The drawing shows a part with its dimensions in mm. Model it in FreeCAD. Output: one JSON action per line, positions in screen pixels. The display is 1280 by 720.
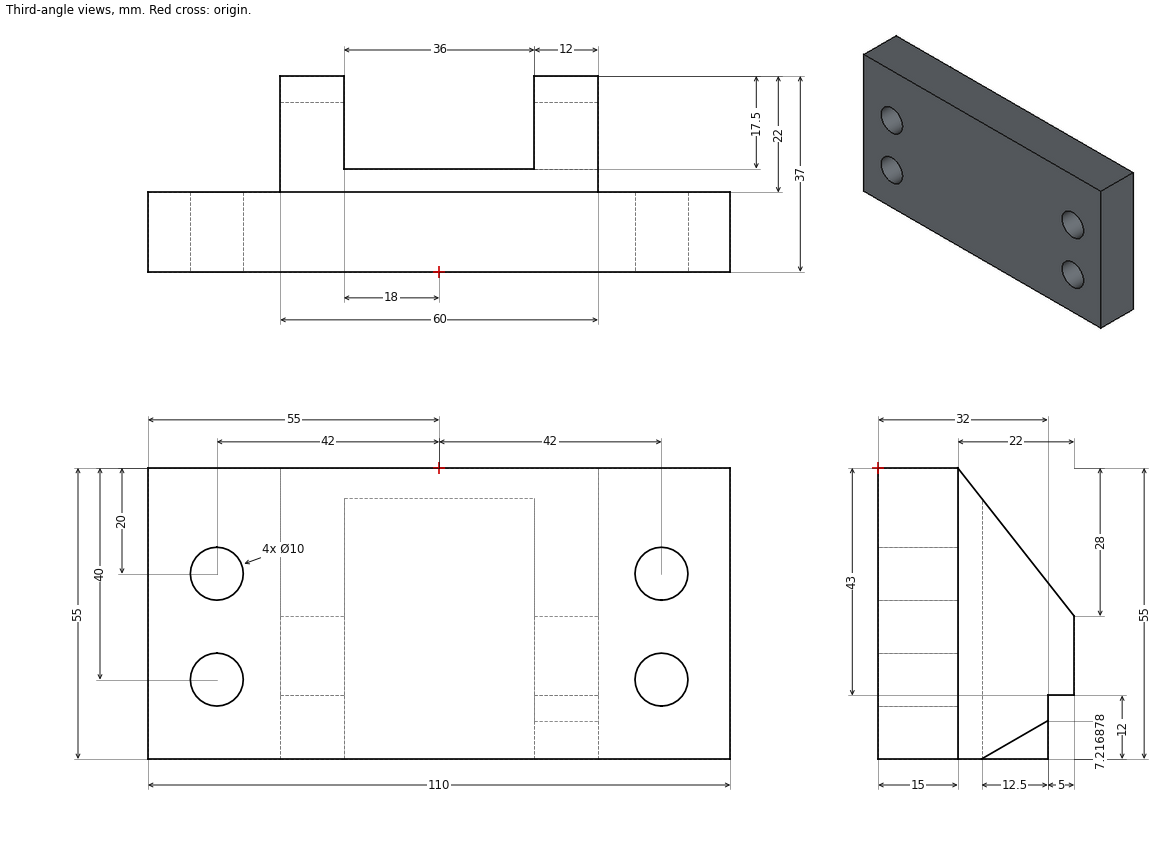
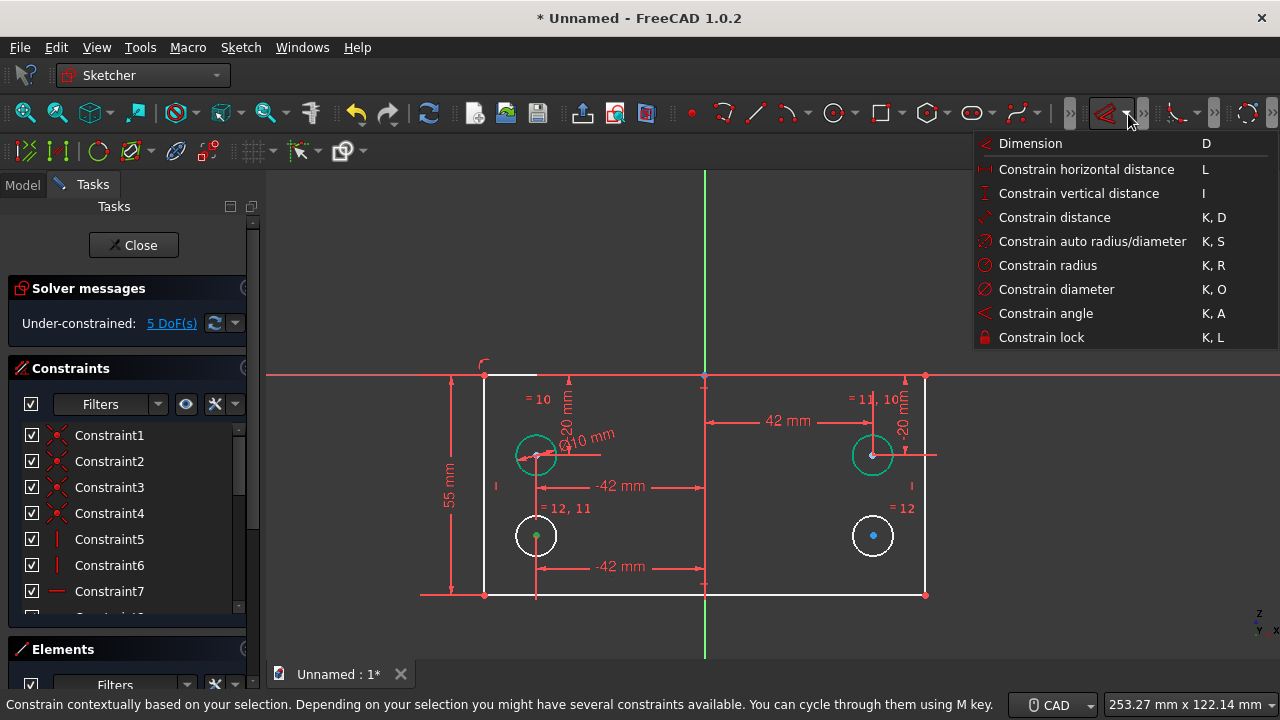
{"action": "left_click", "coordinate": [1126, 193]}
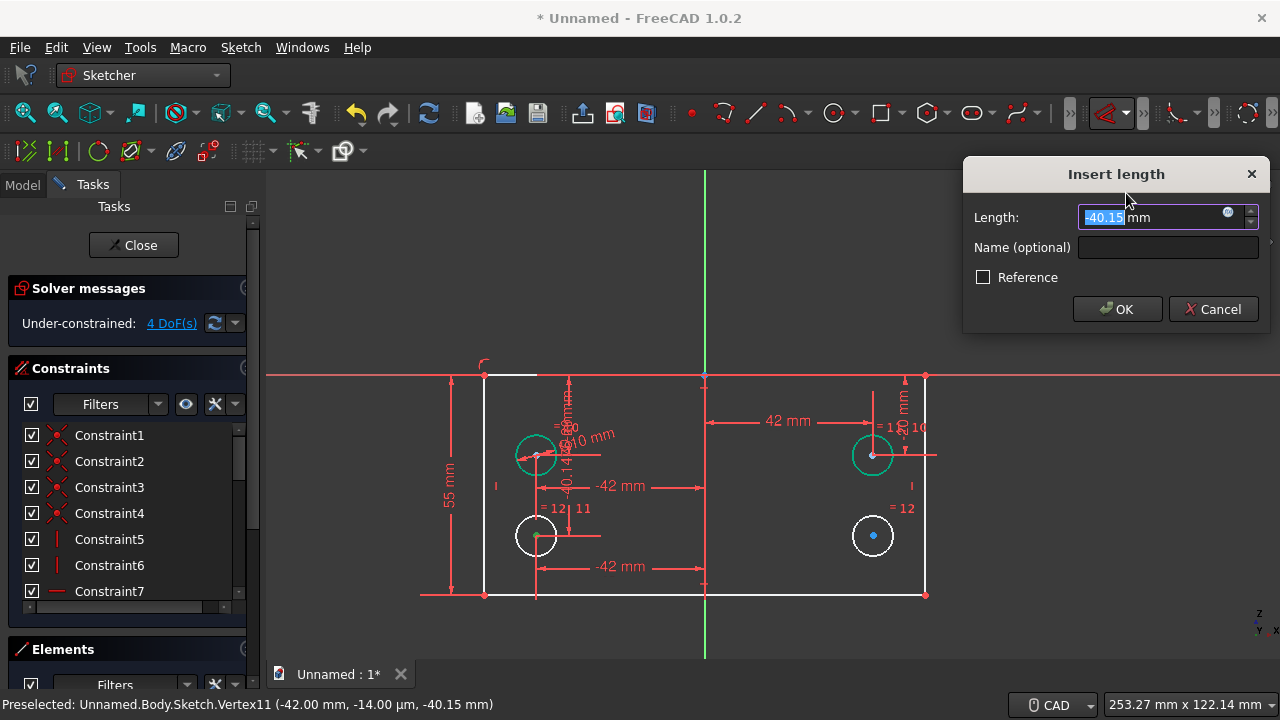
{"action": "type", "text": "-40"}
{"action": "key", "text": "Return"}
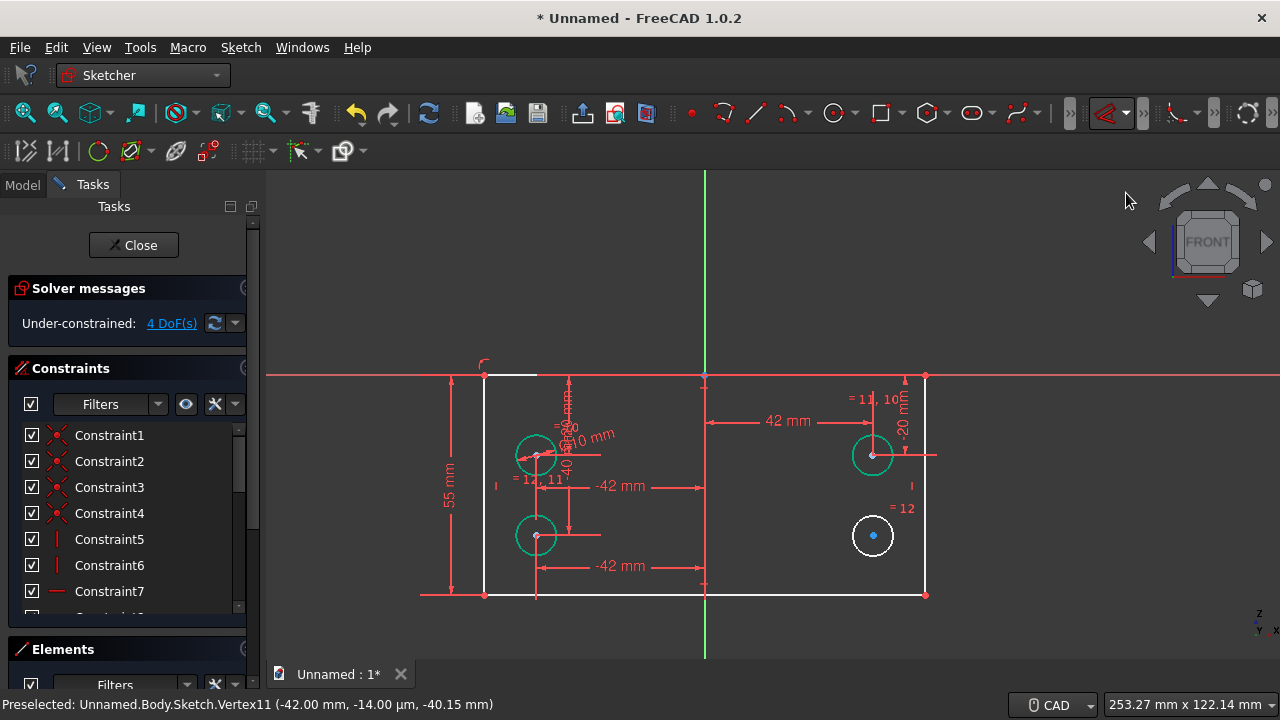
{"action": "left_click", "coordinate": [873, 536]}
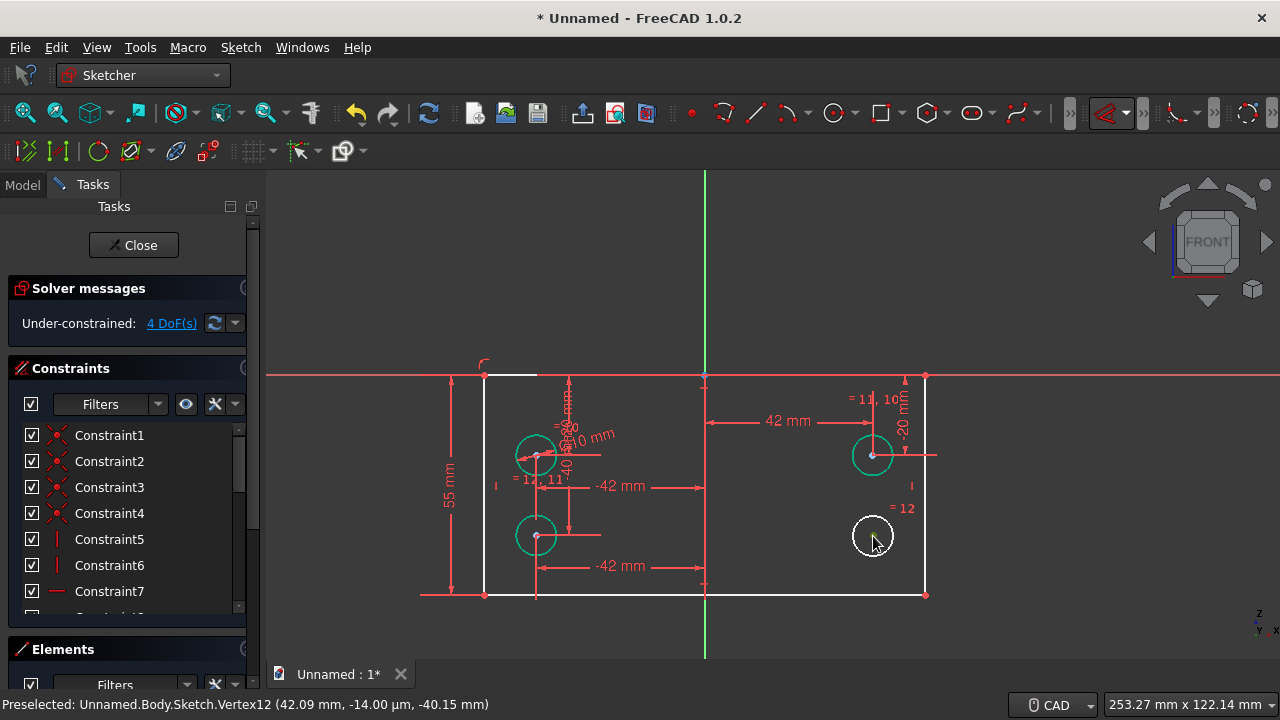
{"action": "key", "text": "l"}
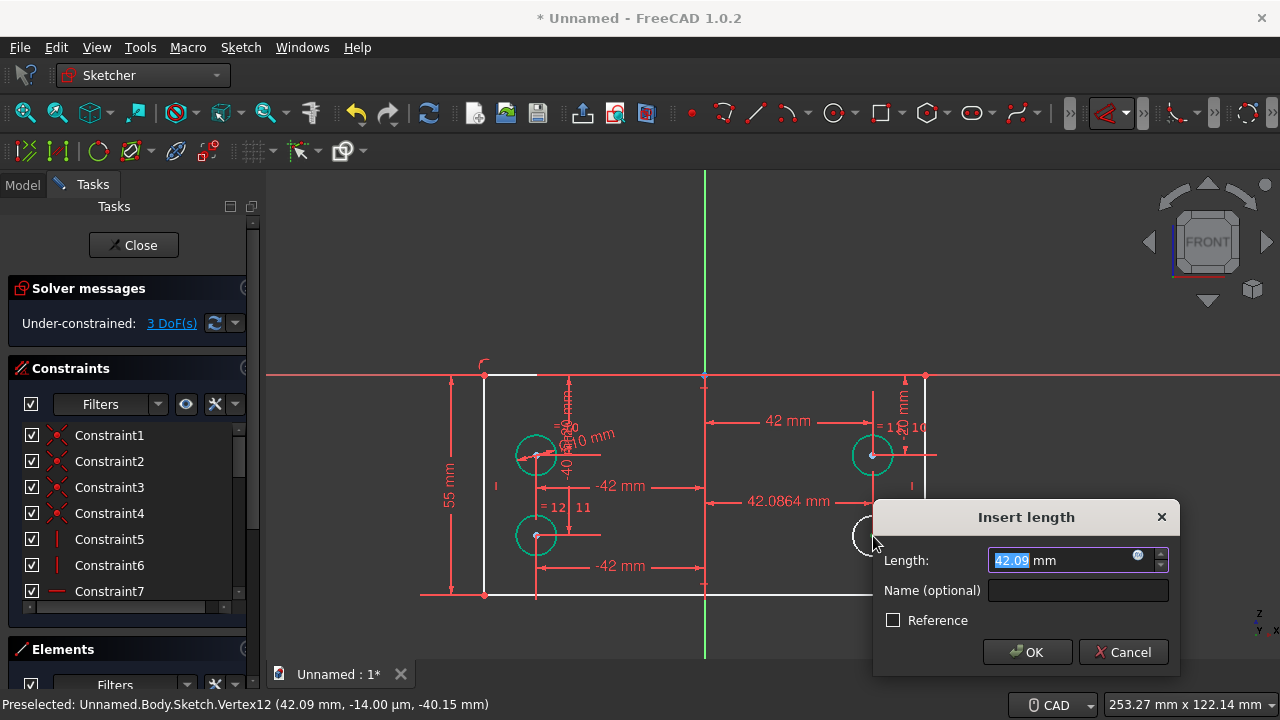
{"action": "type", "text": "42"}
{"action": "key", "text": "Return"}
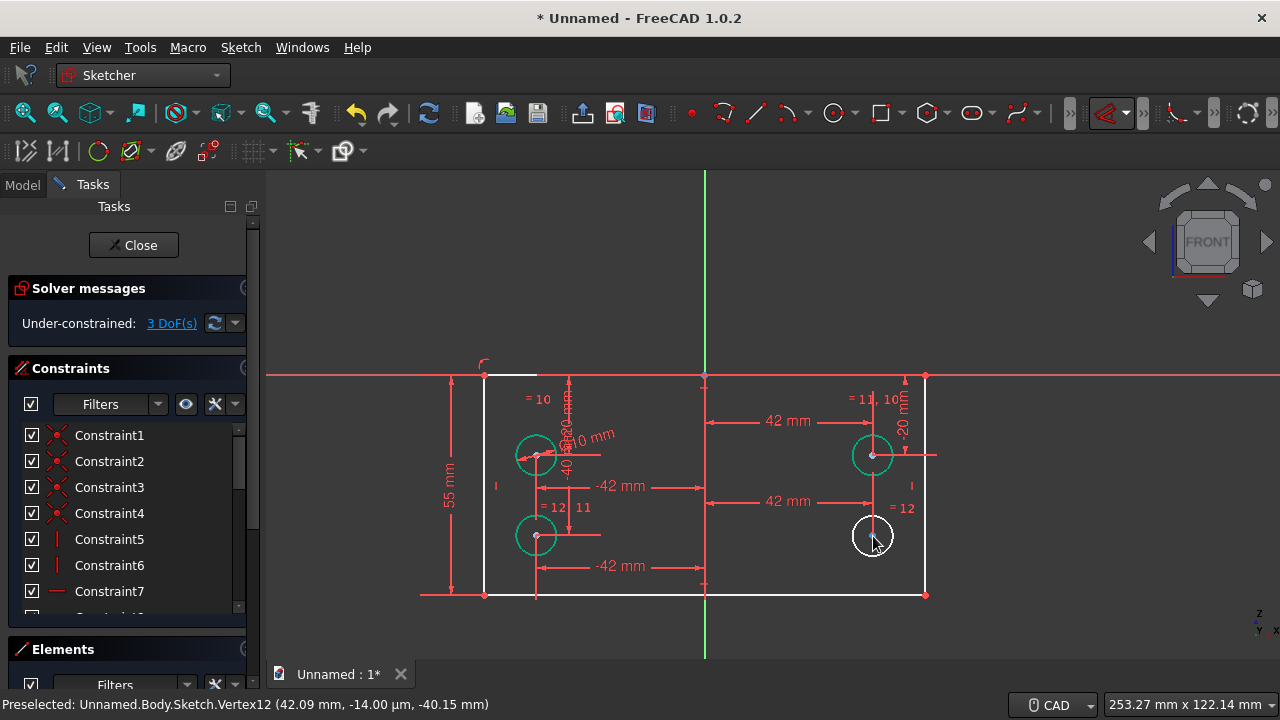
{"action": "left_click", "coordinate": [873, 536]}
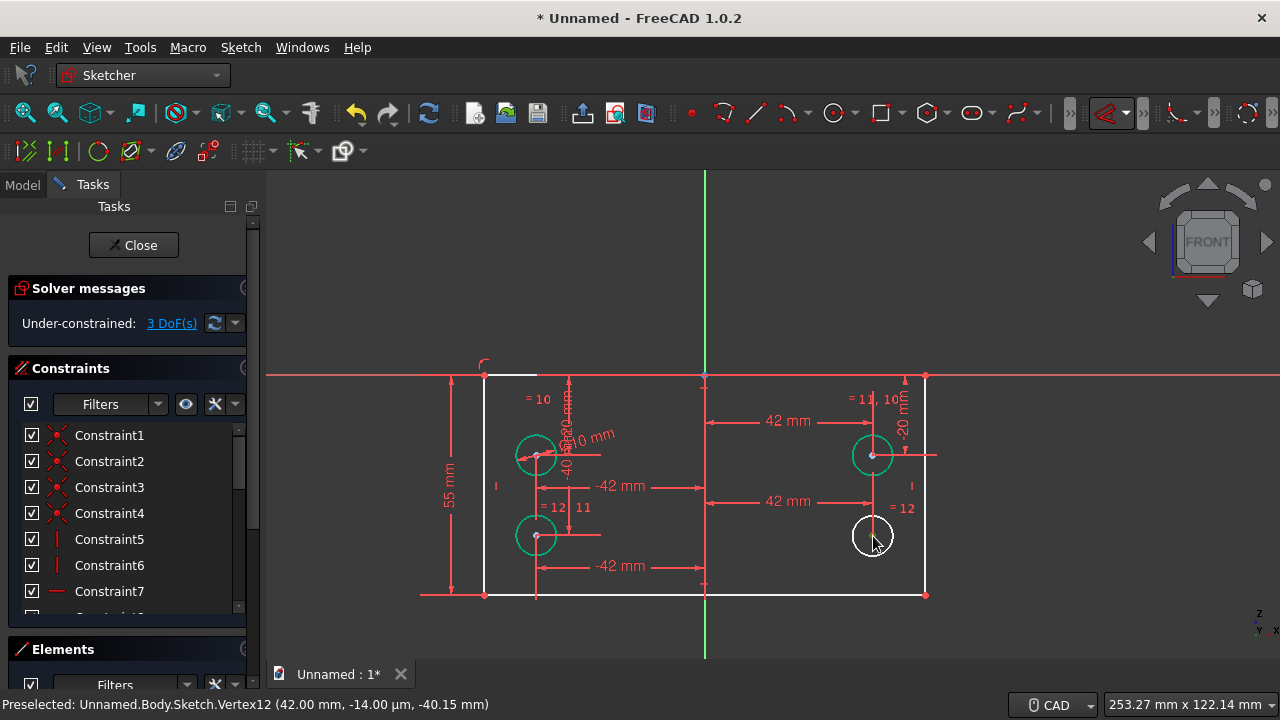
{"action": "key", "text": "i"}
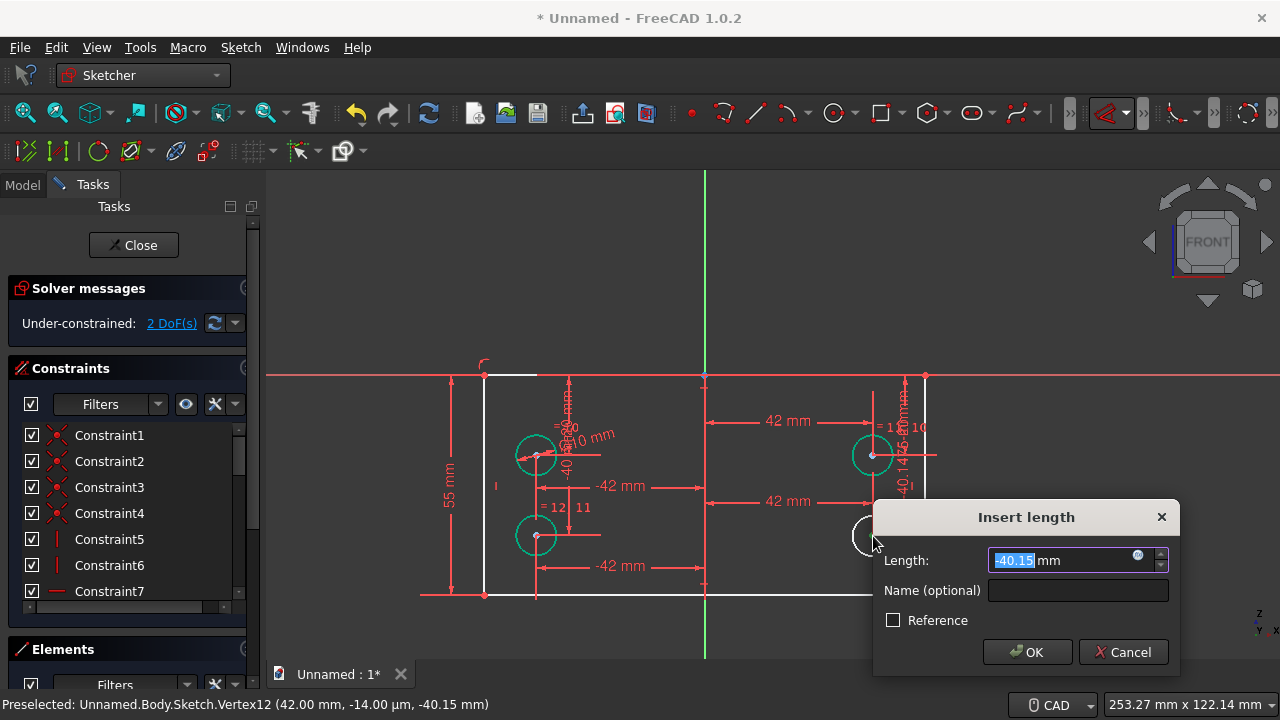
{"action": "type", "text": "-40"}
{"action": "key", "text": "Return"}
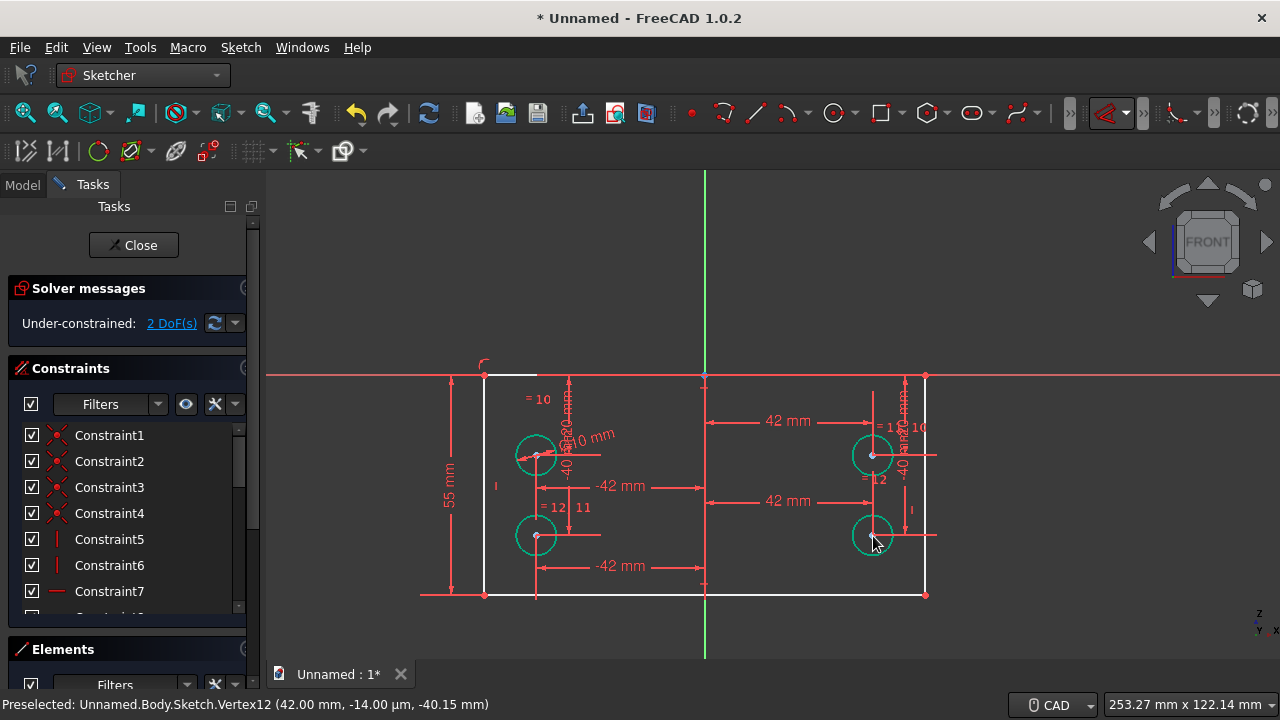
{"action": "left_click", "coordinate": [616, 595]}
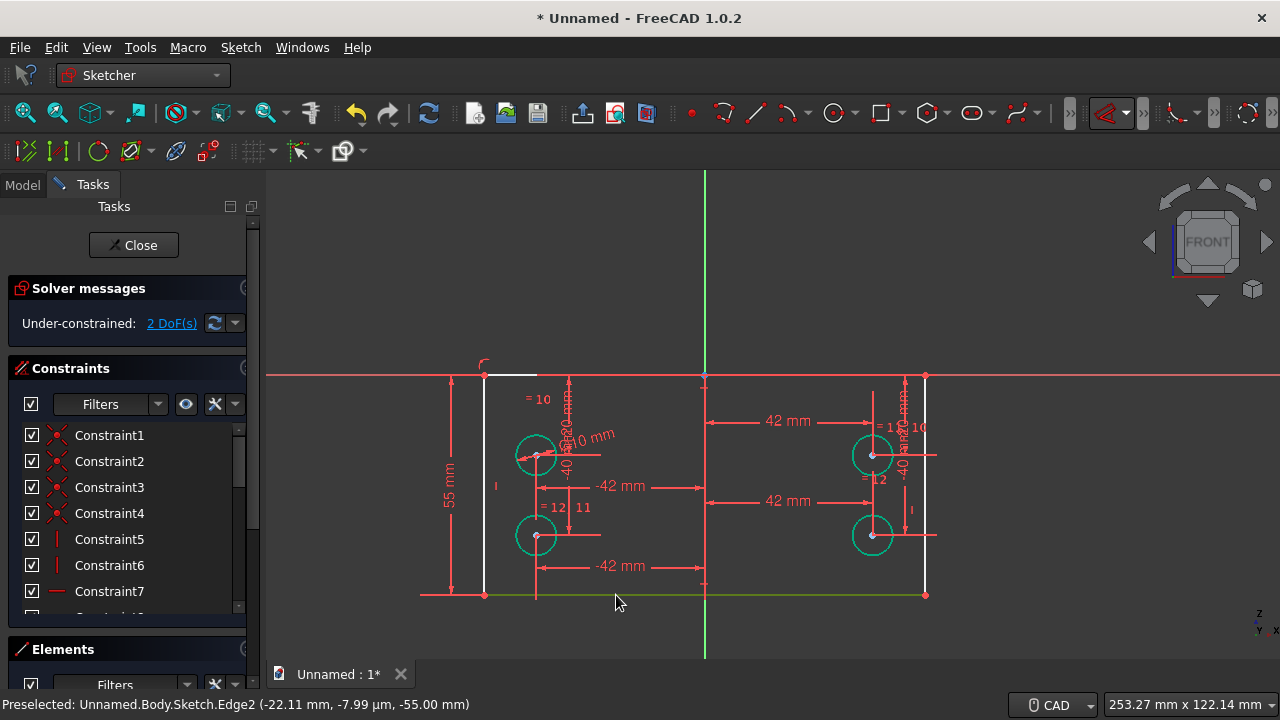
{"action": "left_click", "coordinate": [1128, 114]}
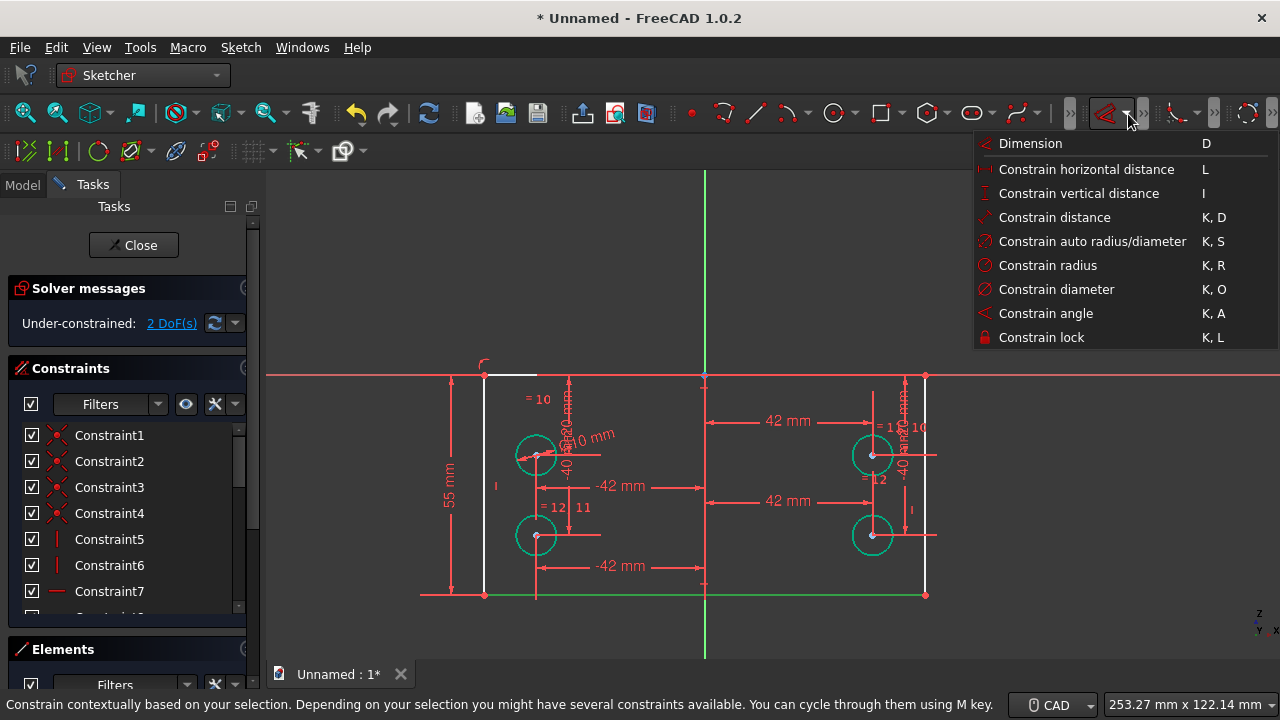
{"action": "left_click", "coordinate": [1126, 169]}